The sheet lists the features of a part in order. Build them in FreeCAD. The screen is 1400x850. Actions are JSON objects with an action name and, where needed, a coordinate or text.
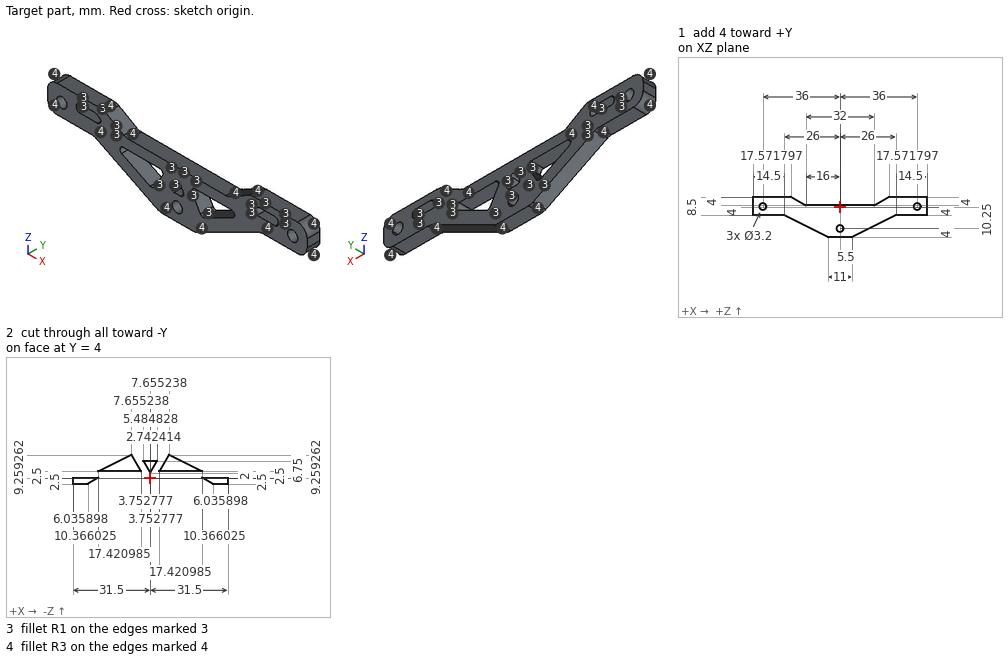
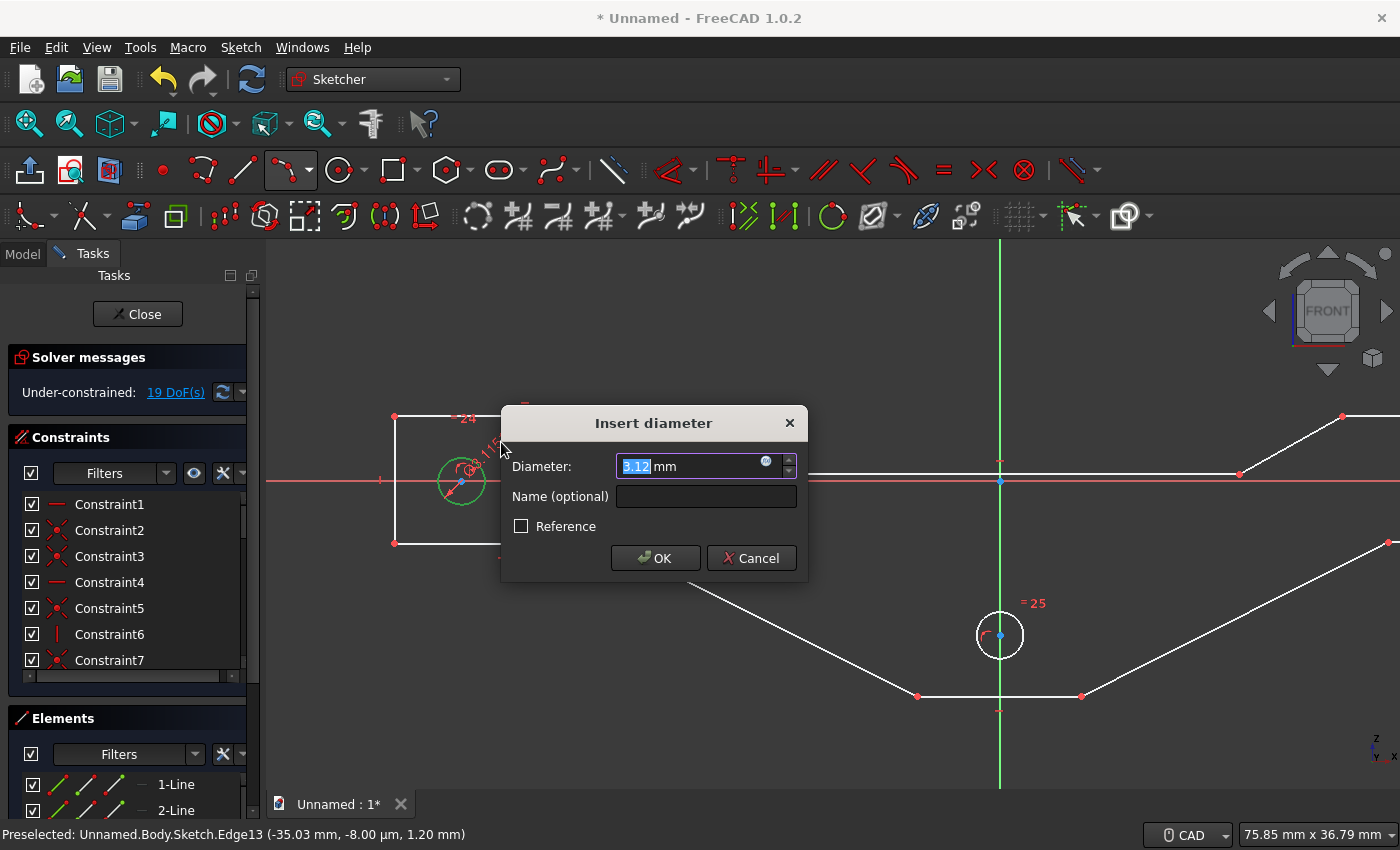
{"action": "type", "text": "3.2"}
{"action": "key", "text": "Return"}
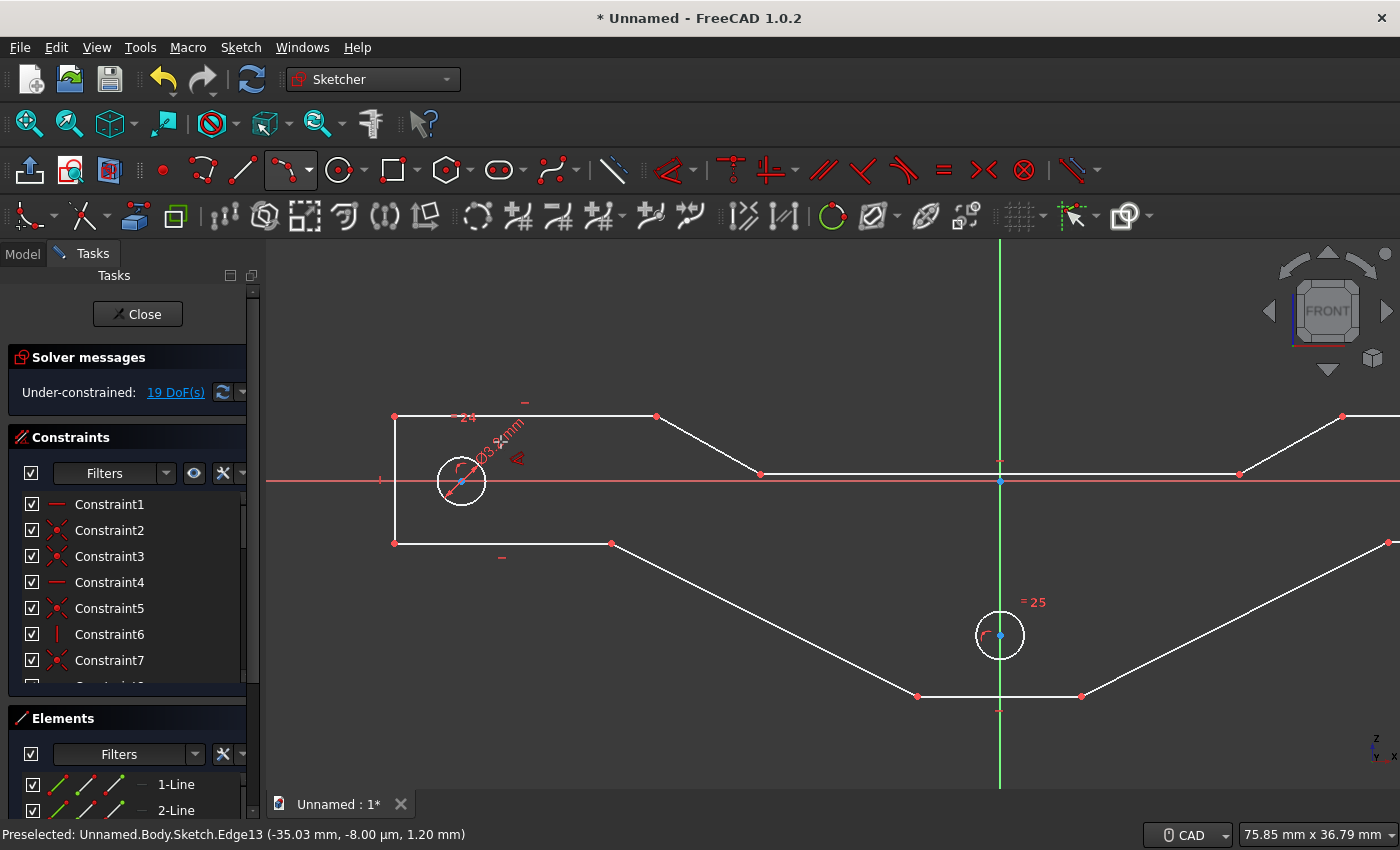
{"action": "left_click", "coordinate": [1032, 697]}
{"action": "left_click", "coordinate": [962, 731]}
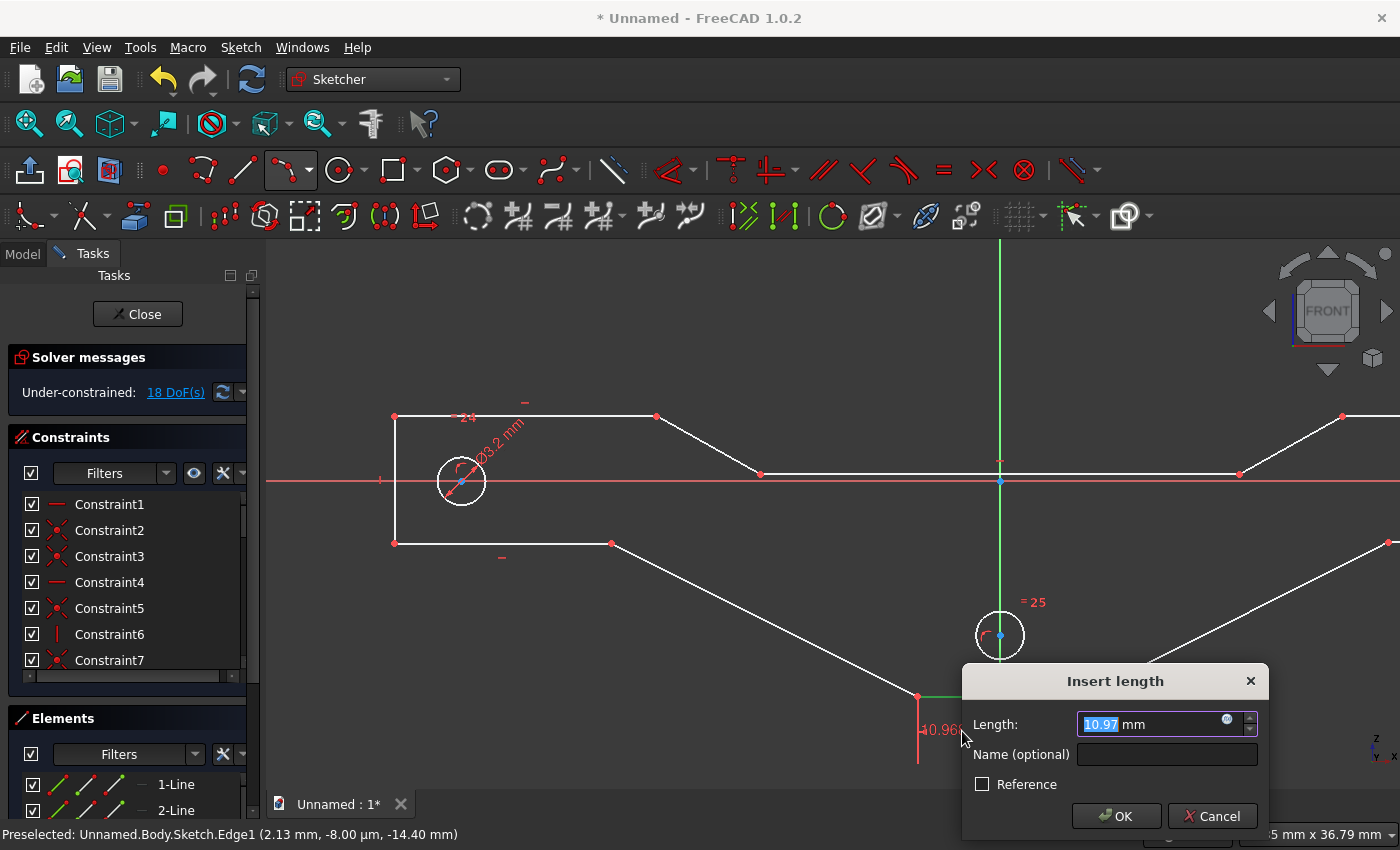
{"action": "type", "text": "11"}
{"action": "key", "text": "Return"}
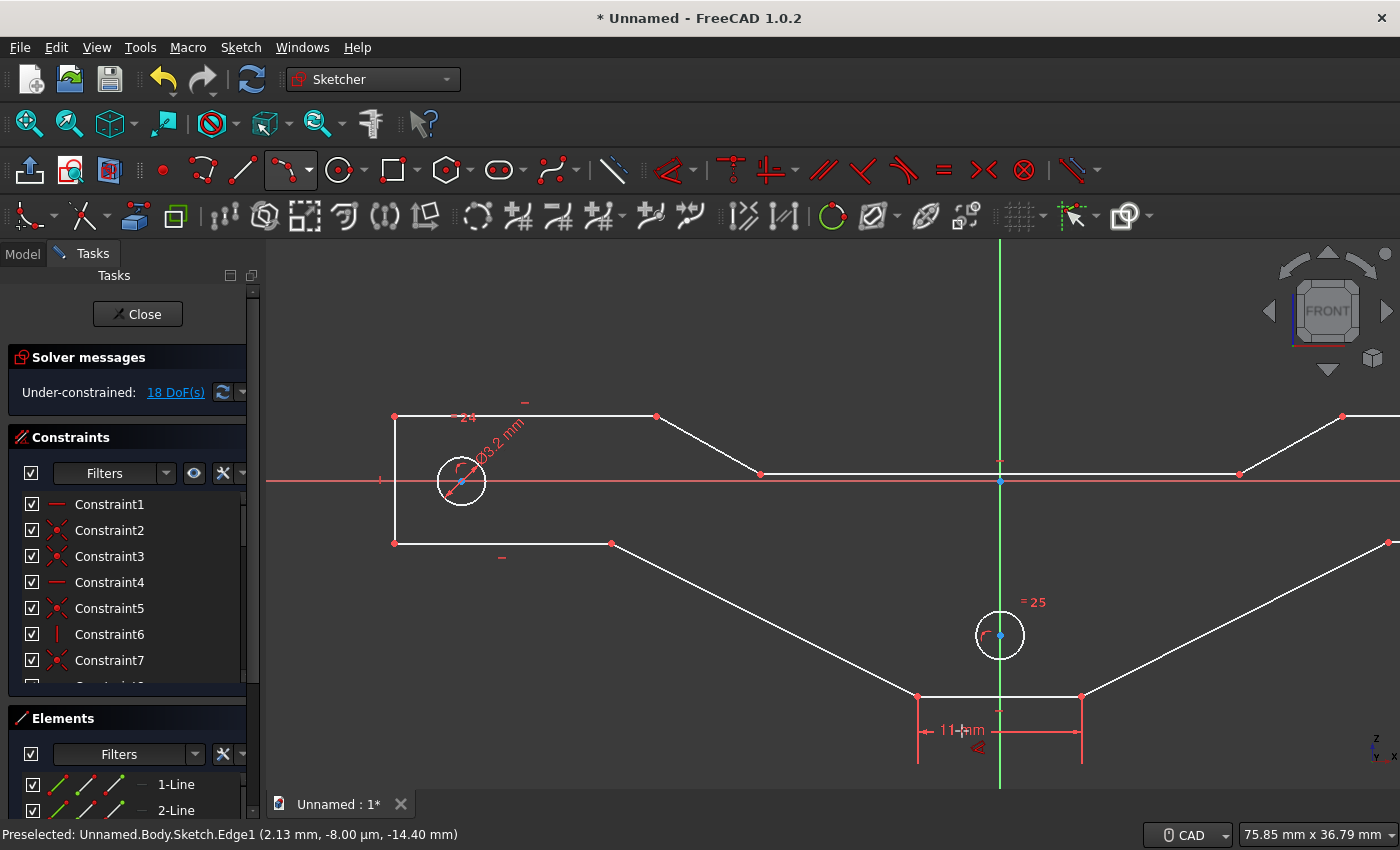
{"action": "scroll", "coordinate": [904, 474], "scroll_direction": "up", "scroll_amount": 4}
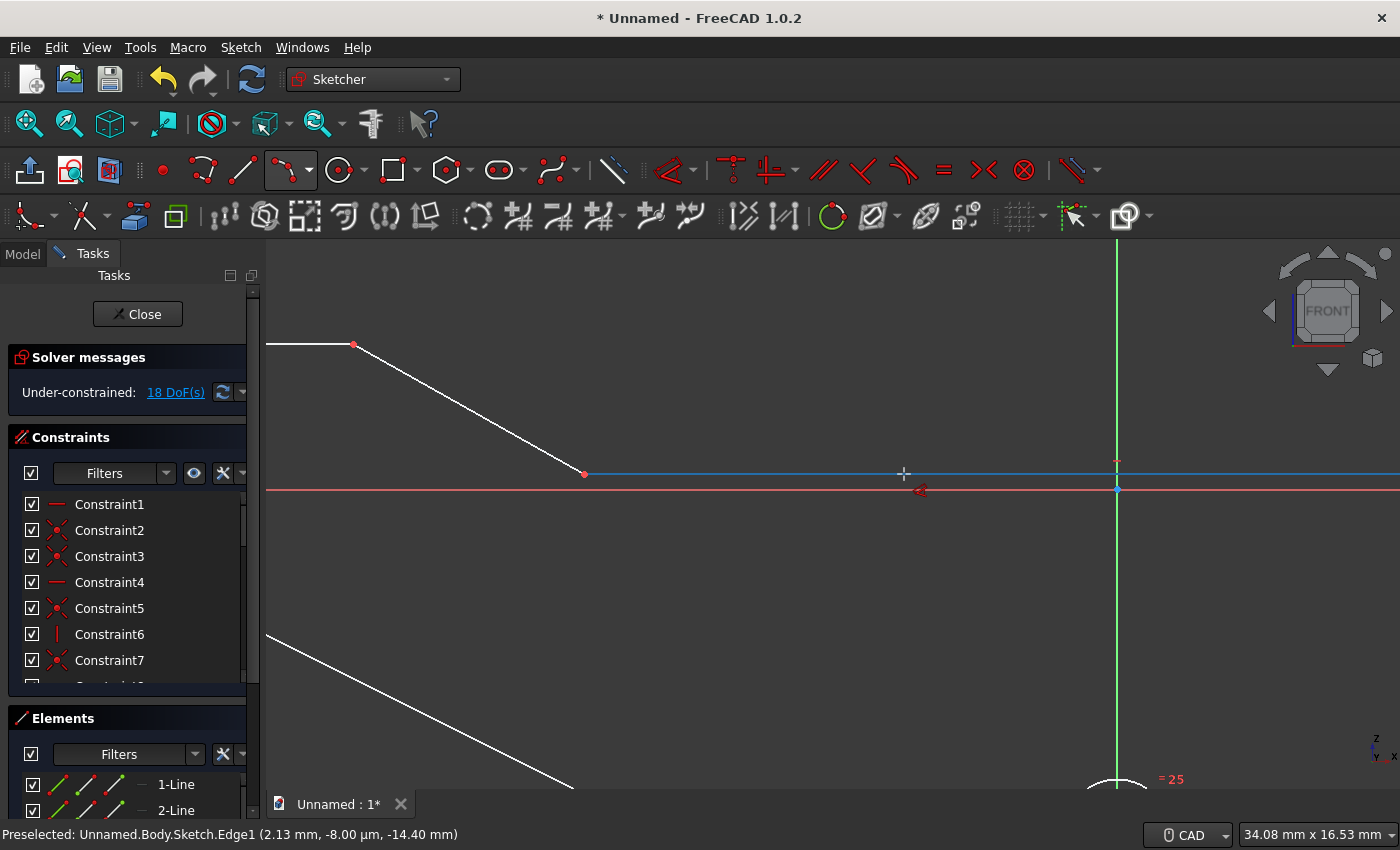
{"action": "left_click", "coordinate": [904, 474]}
{"action": "left_click", "coordinate": [910, 440]}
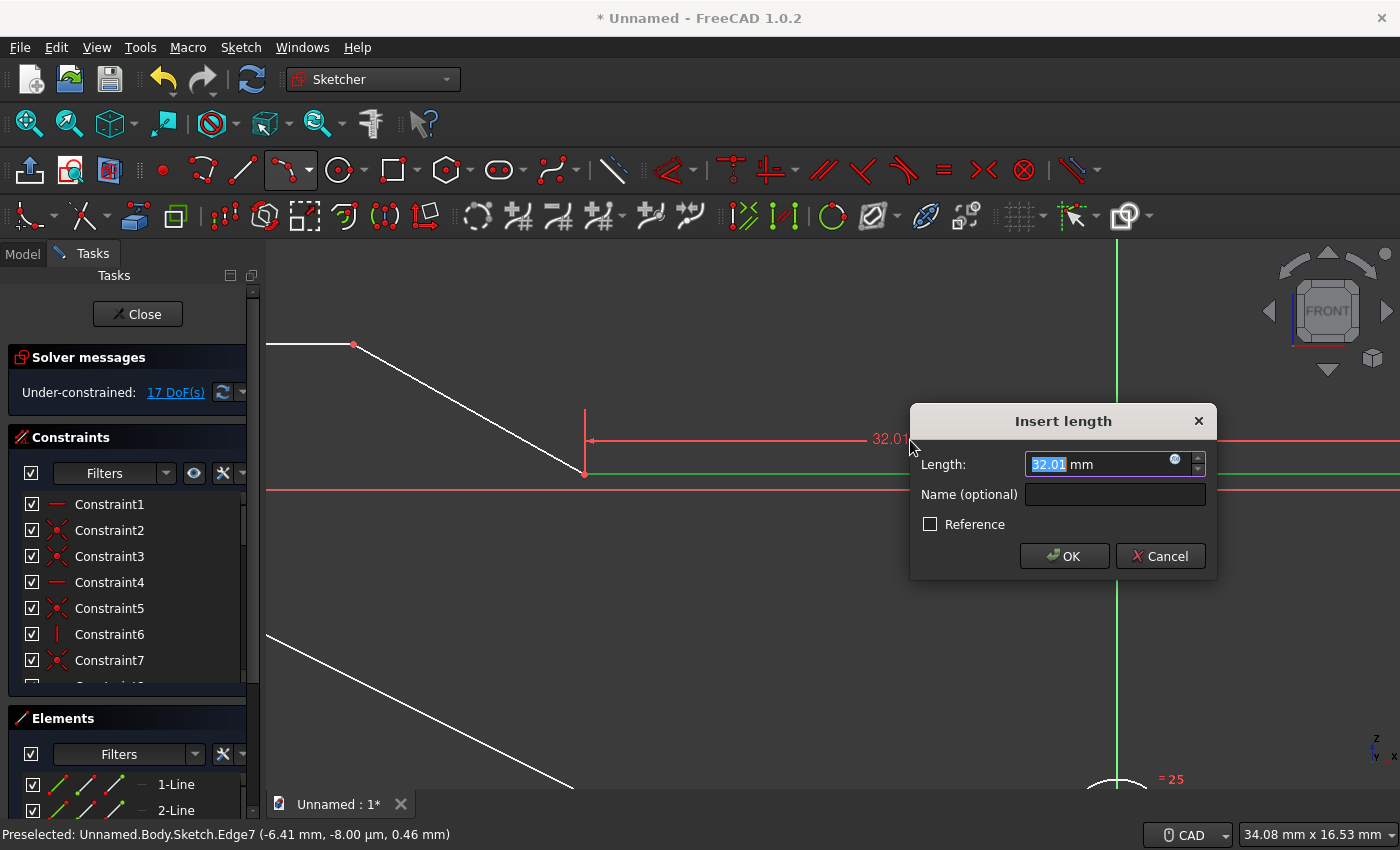
{"action": "type", "text": "32"}
{"action": "key", "text": "Return"}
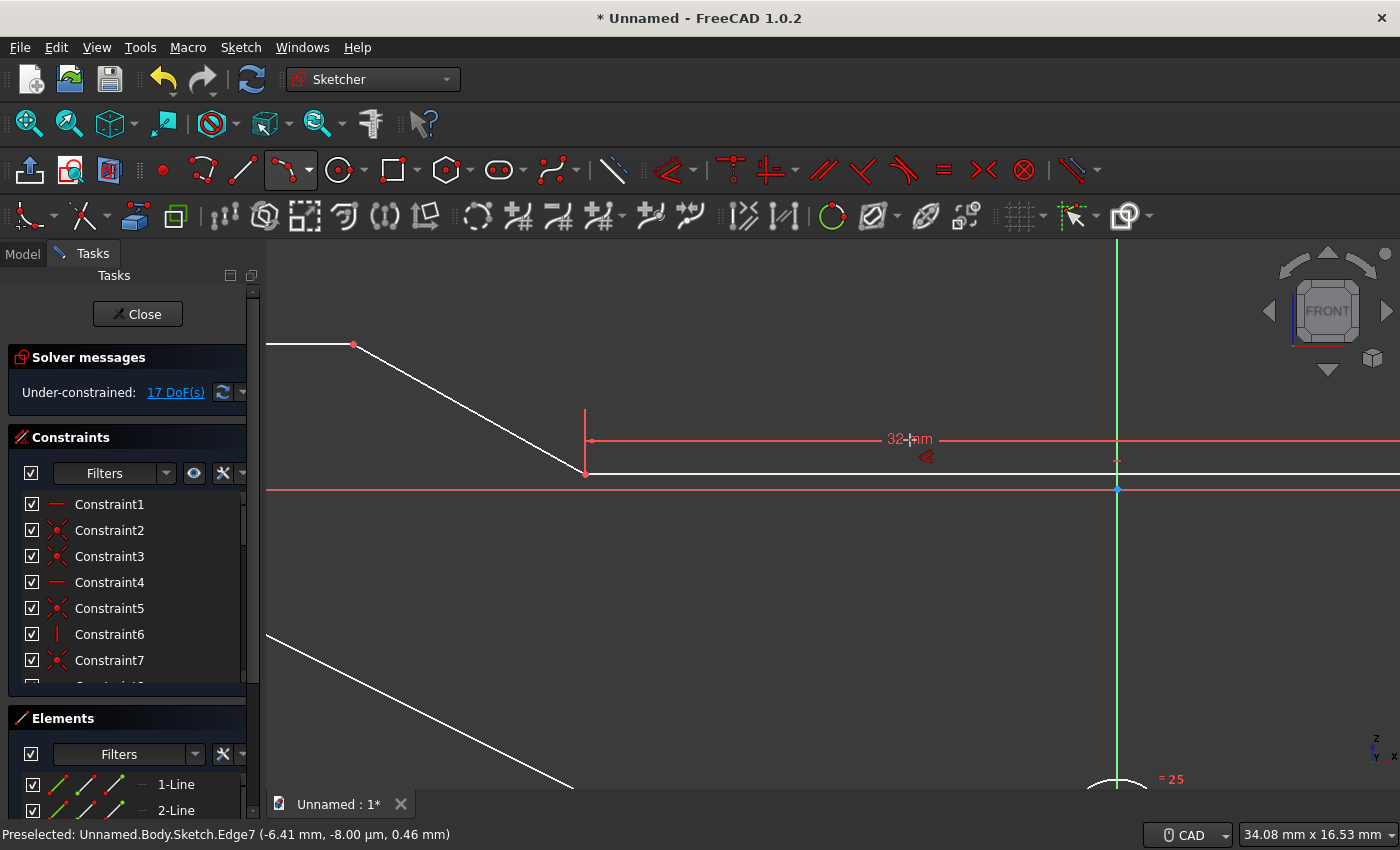
{"action": "scroll", "coordinate": [649, 469], "scroll_direction": "down", "scroll_amount": 7}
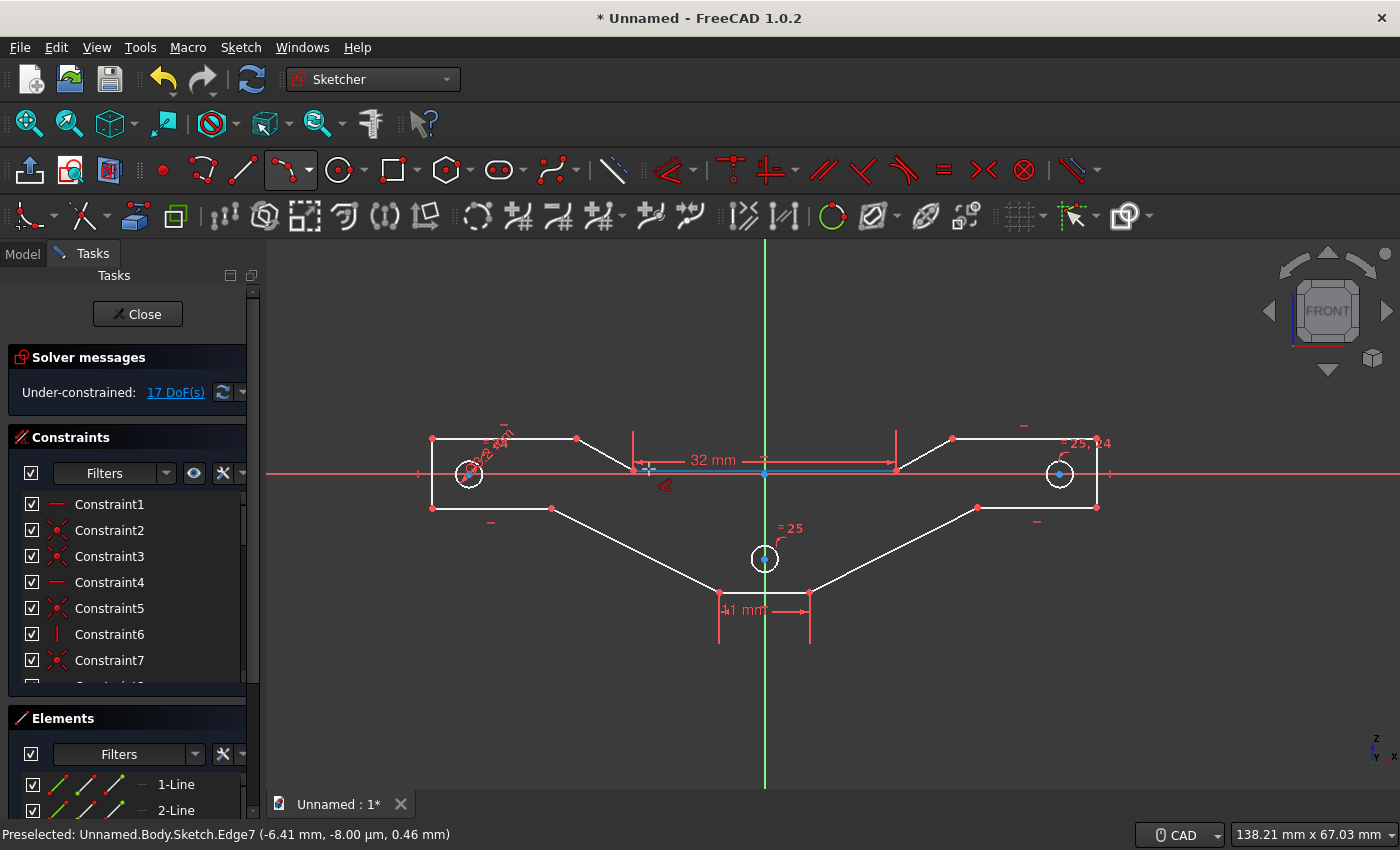
{"action": "left_click", "coordinate": [551, 509]}
{"action": "left_click", "coordinate": [517, 492]}